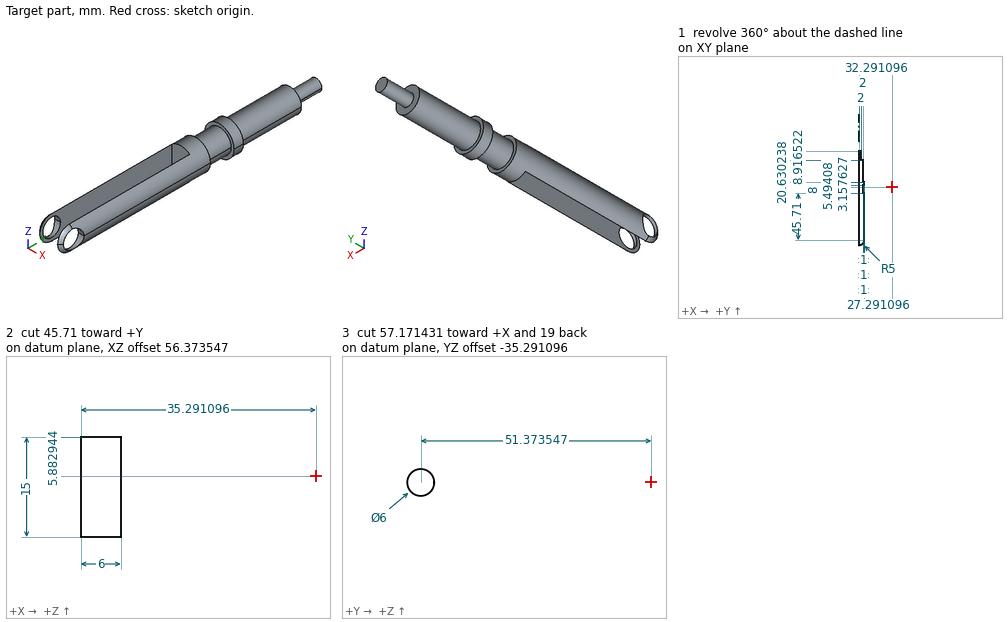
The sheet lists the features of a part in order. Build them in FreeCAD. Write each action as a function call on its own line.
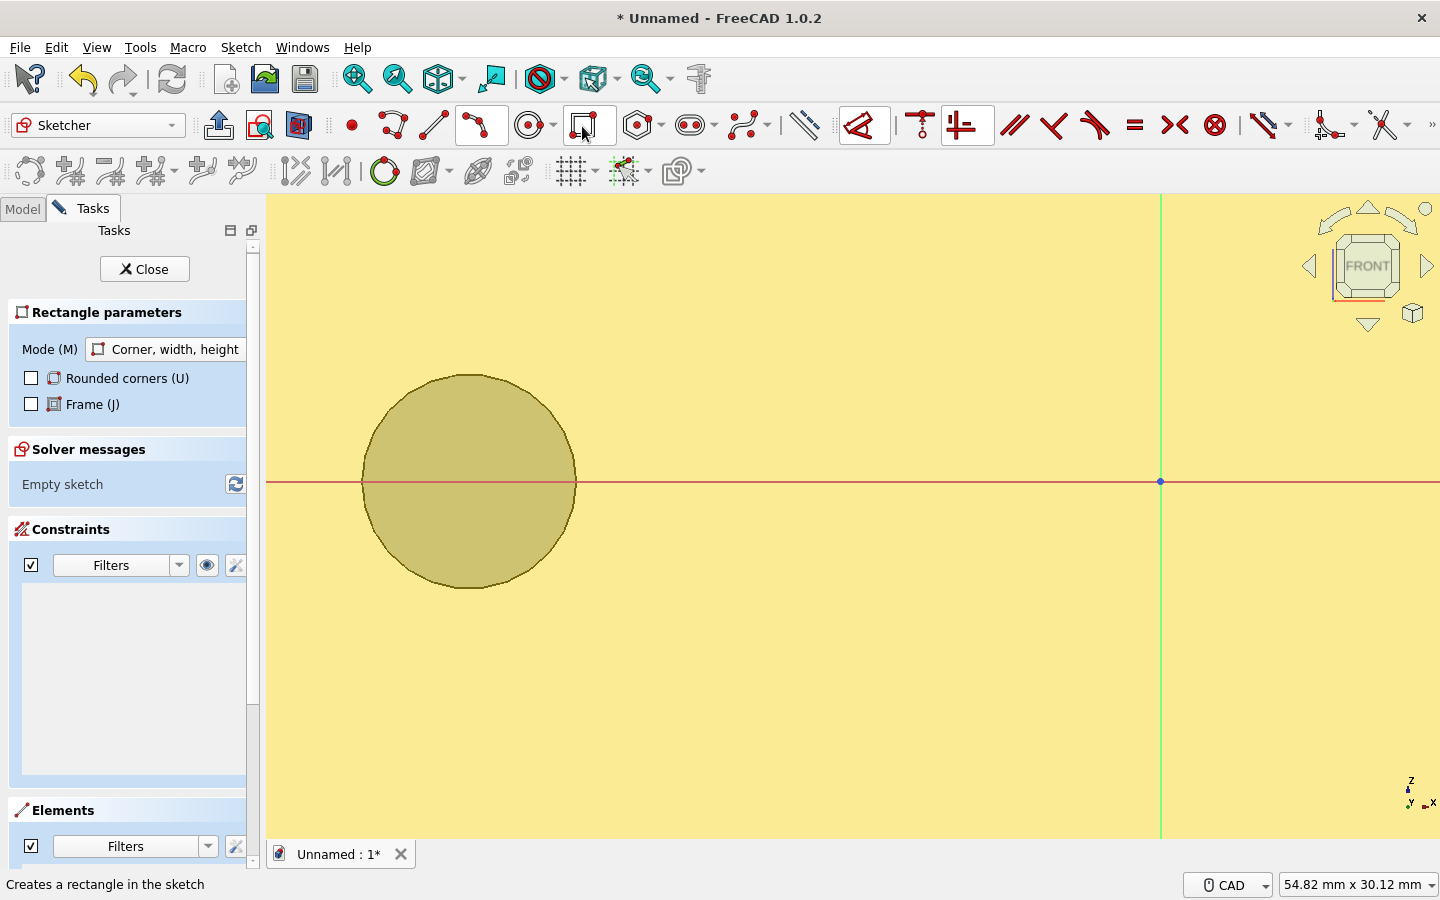
click(405, 356)
click(533, 677)
key(Escape)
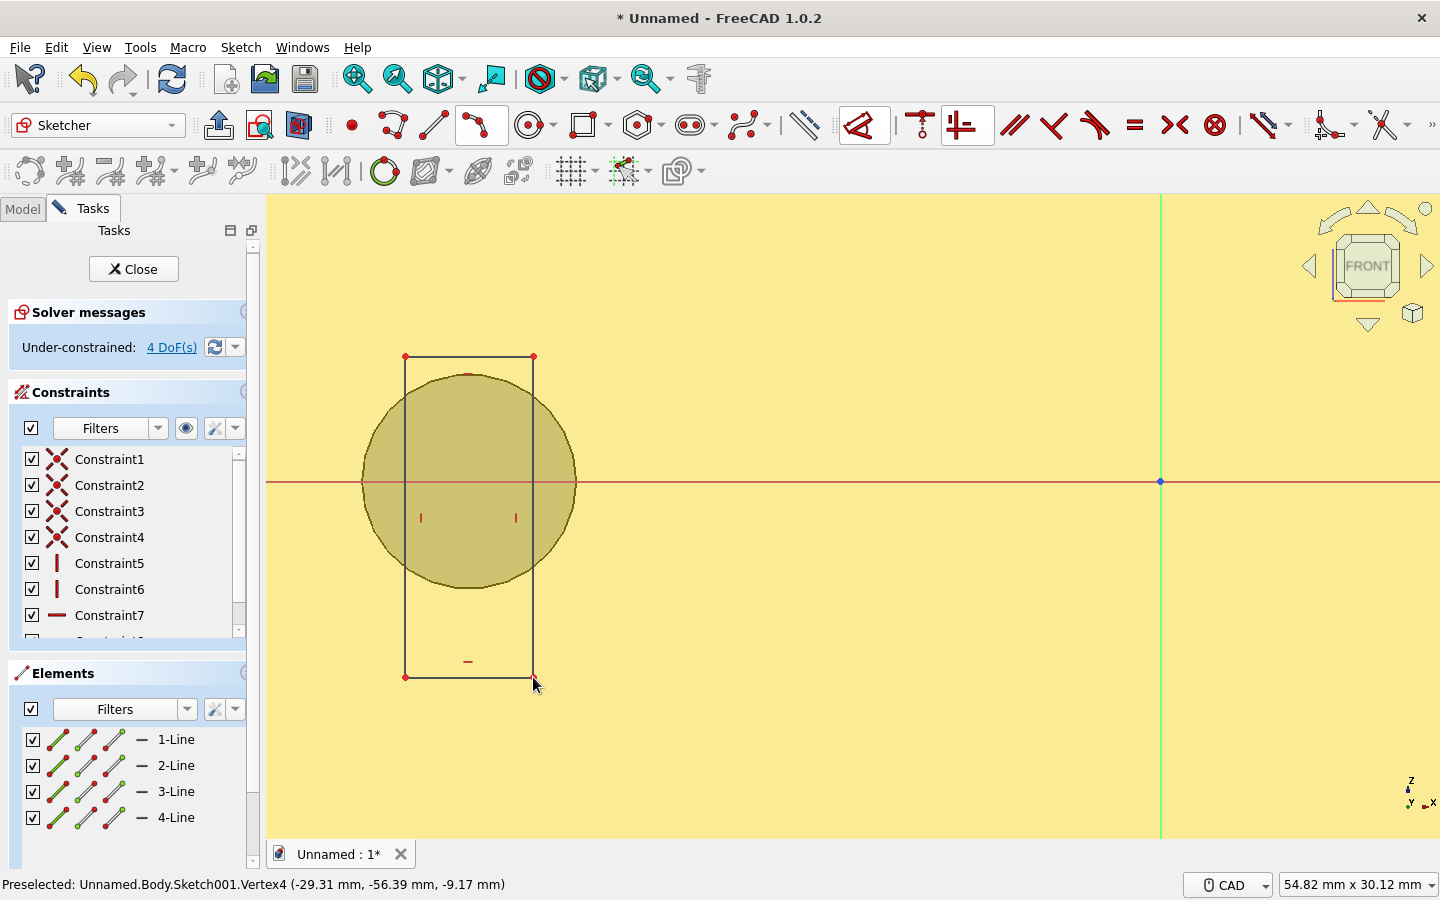
click(443, 678)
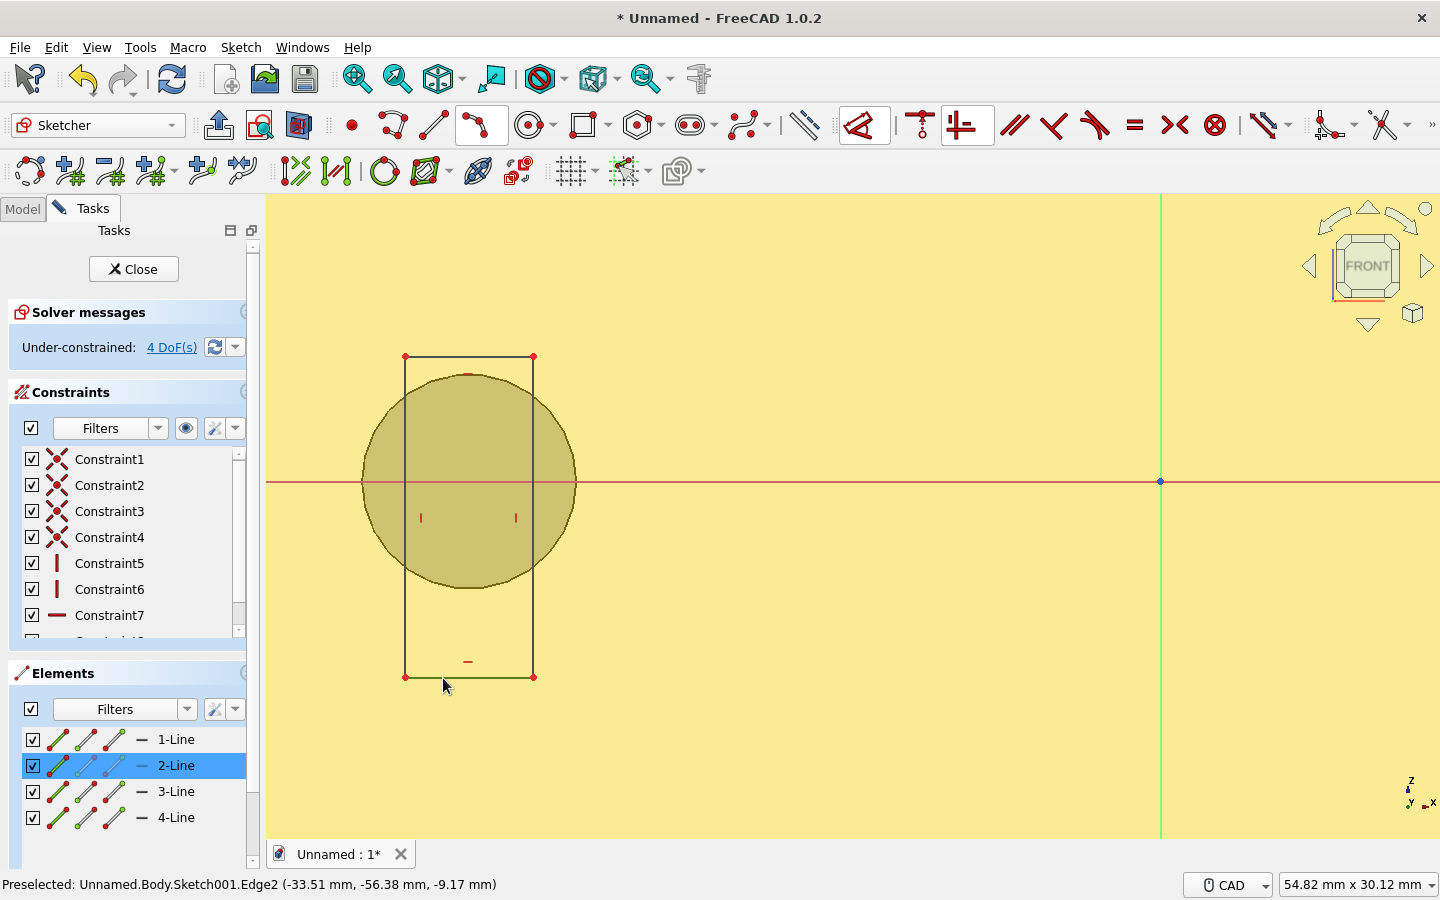
key(l)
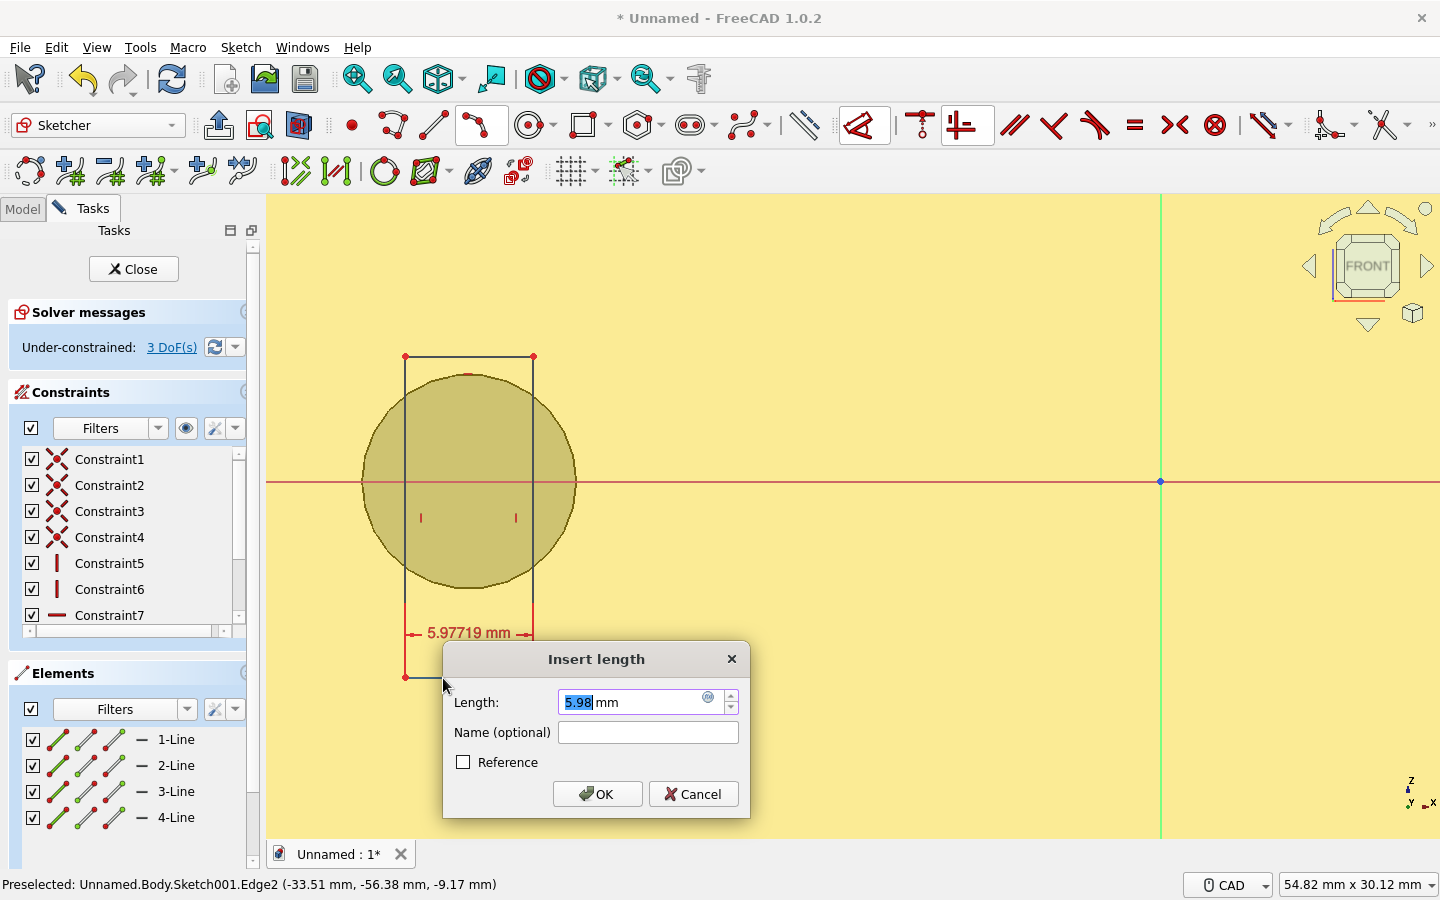
text(6)
key(Return)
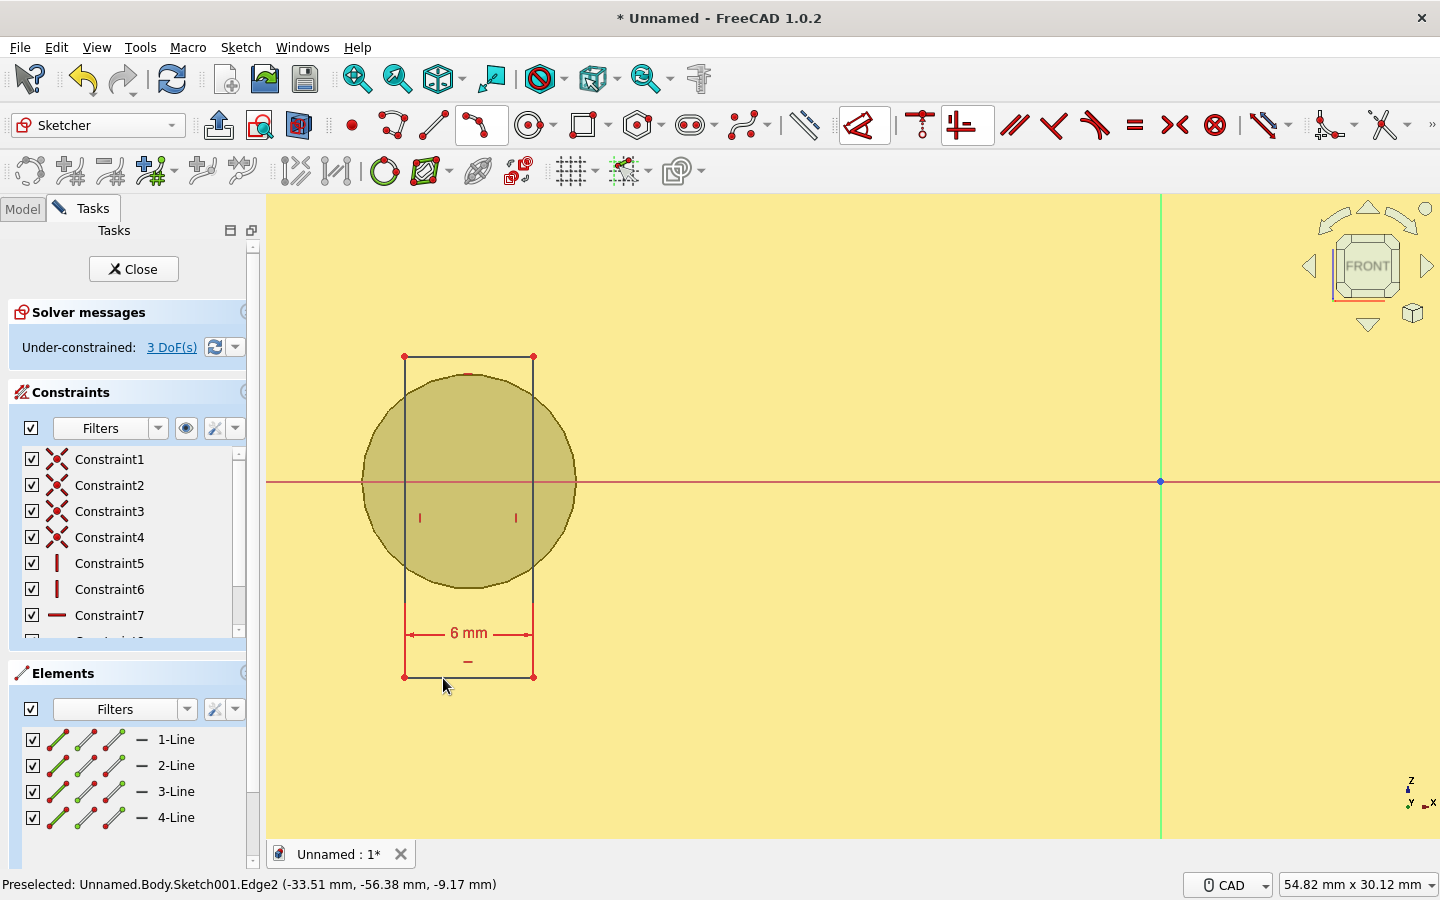
click(405, 453)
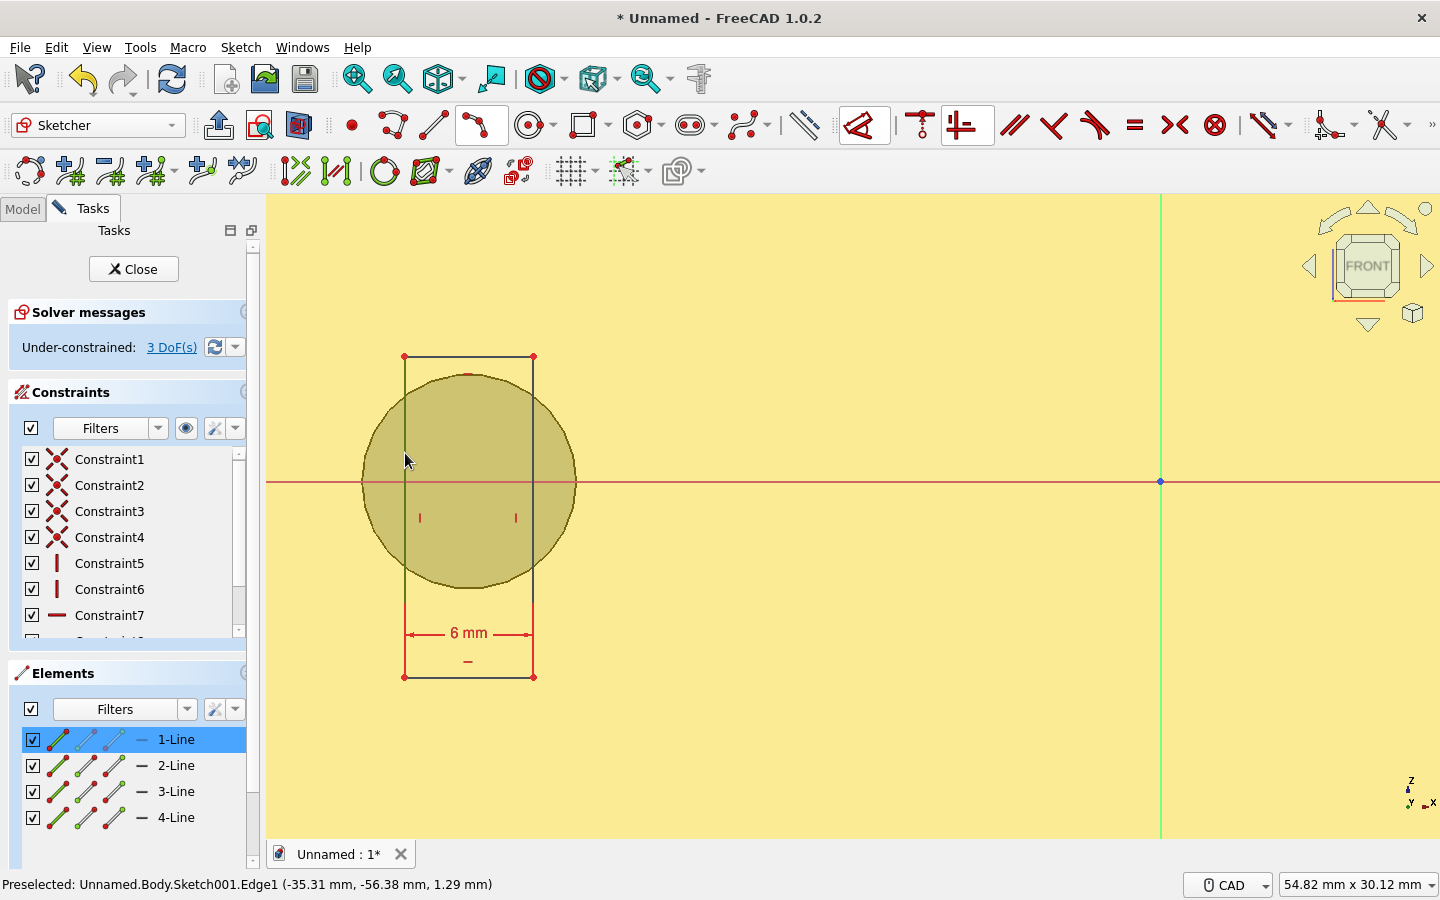
click(884, 126)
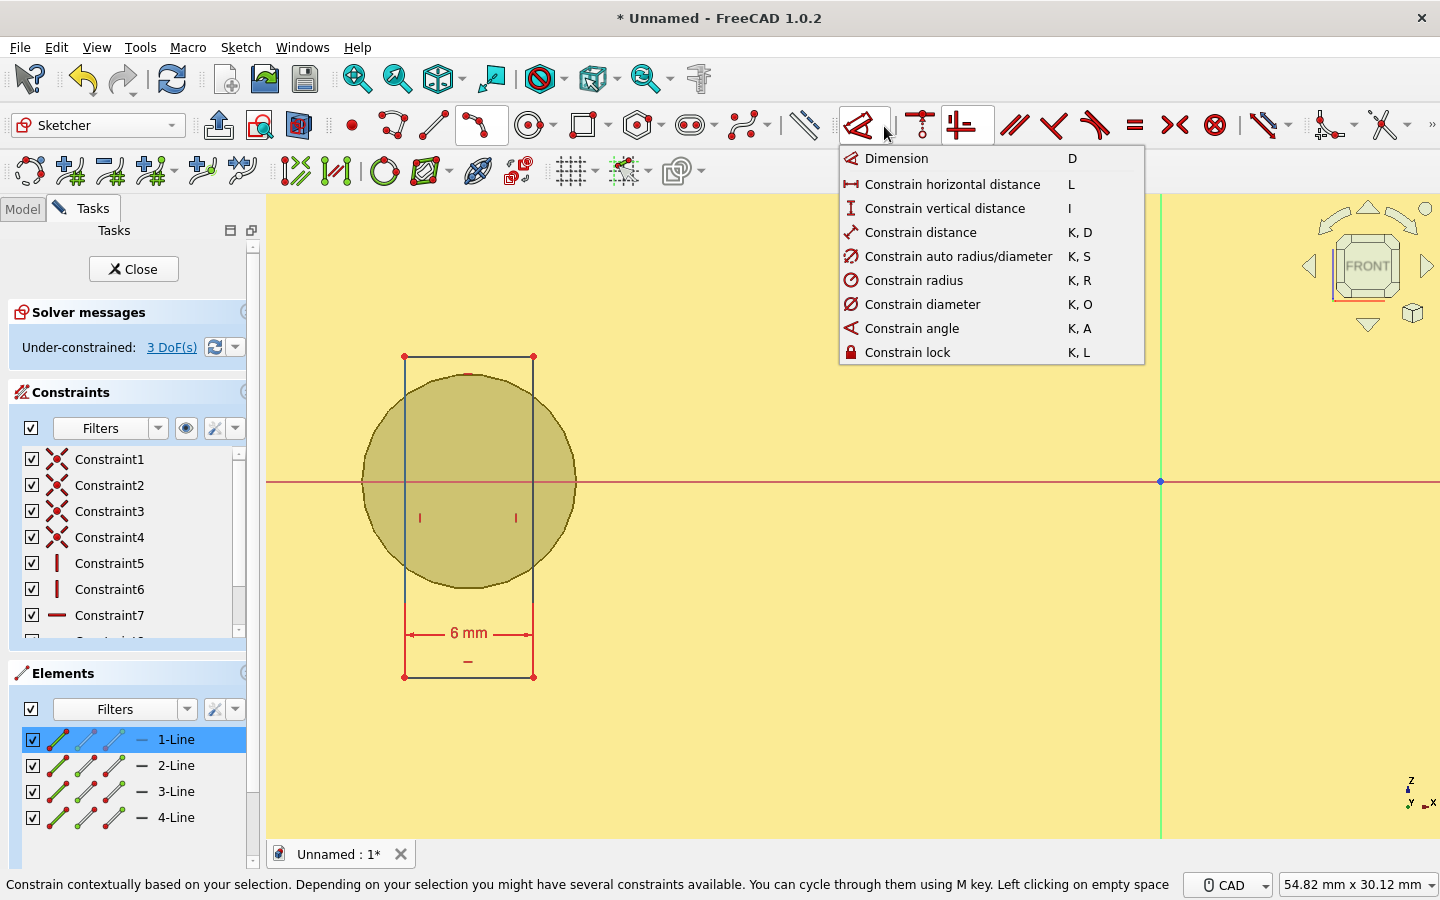
click(992, 208)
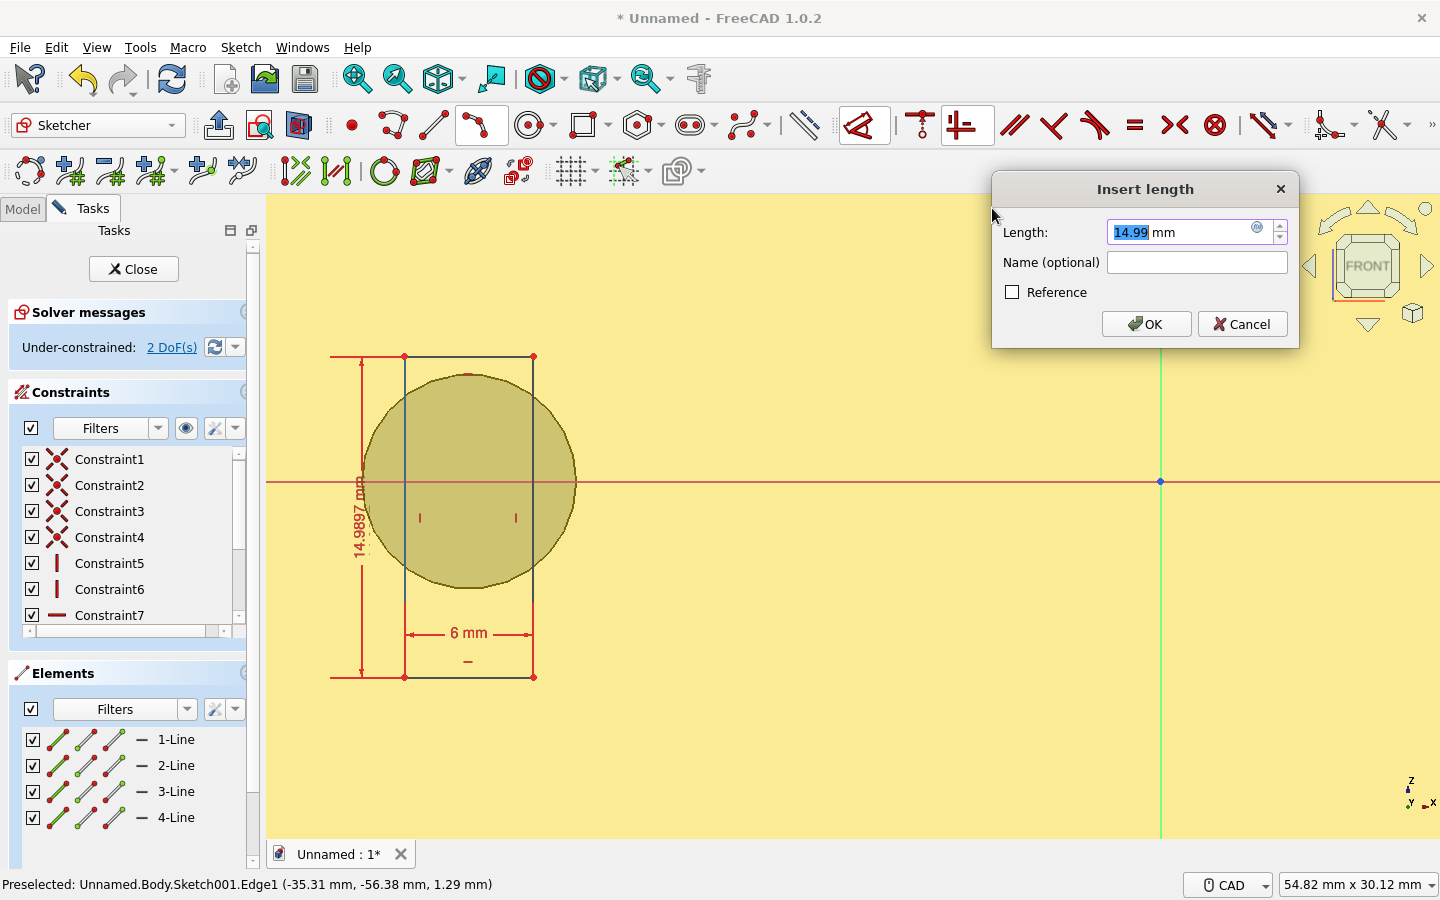
text(15)
key(Return)